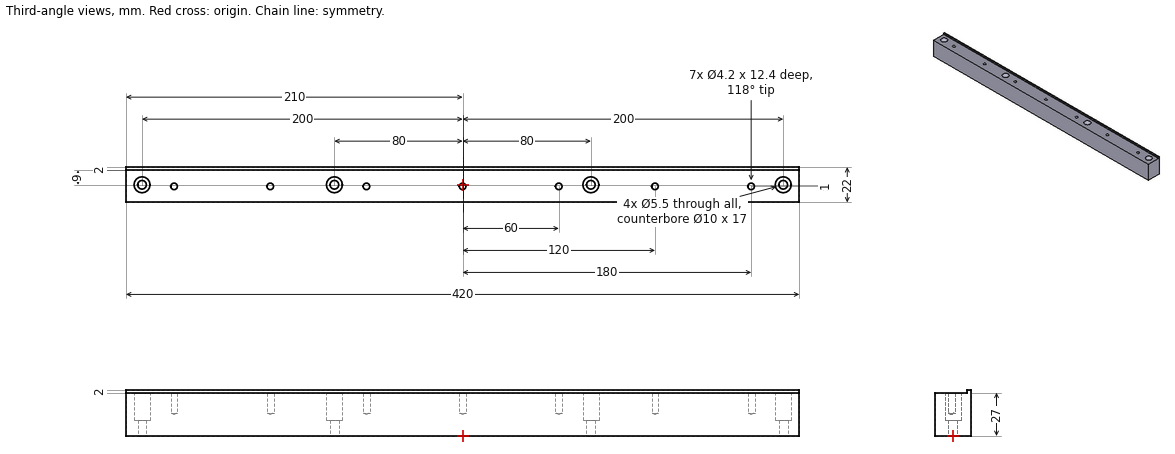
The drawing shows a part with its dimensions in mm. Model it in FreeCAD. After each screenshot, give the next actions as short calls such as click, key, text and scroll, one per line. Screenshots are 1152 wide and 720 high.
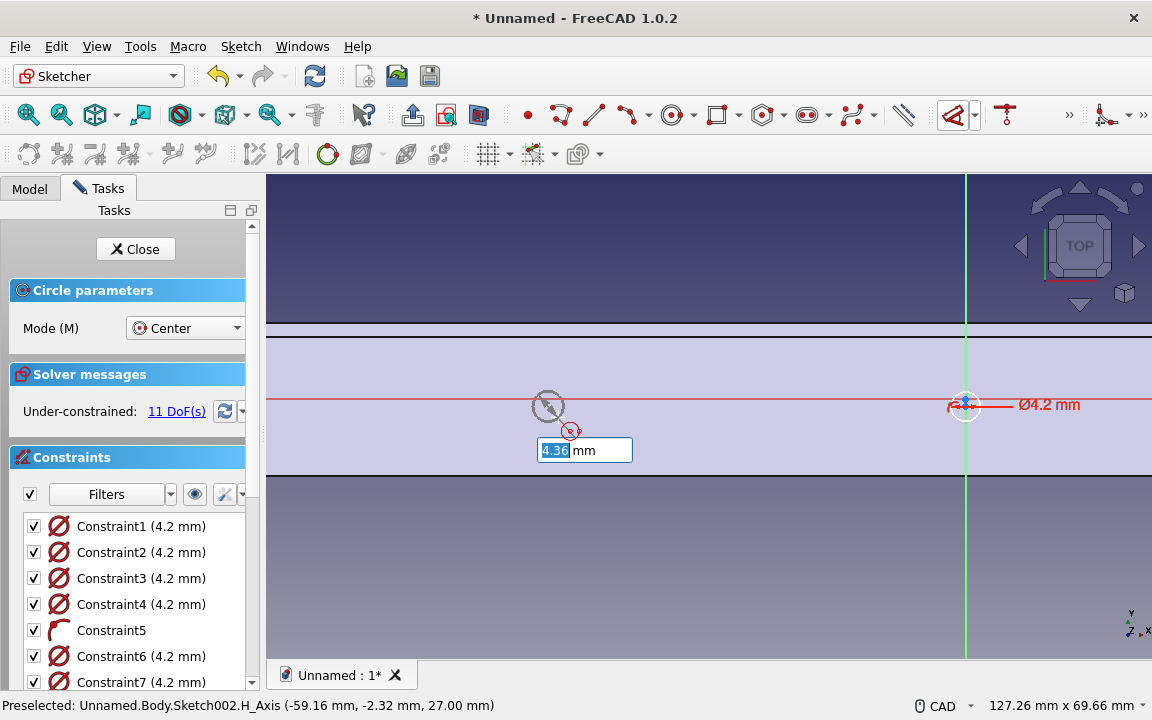
text(4.2)
key(Return)
key(Escape)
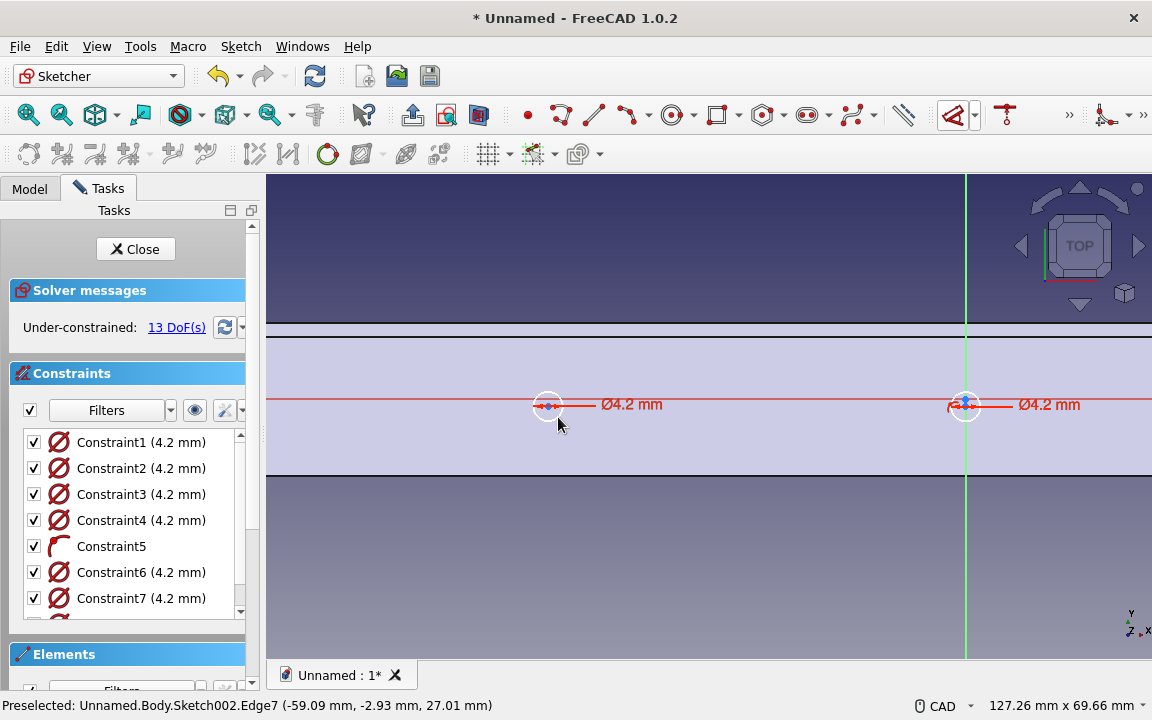
scroll(558, 419, down, 8)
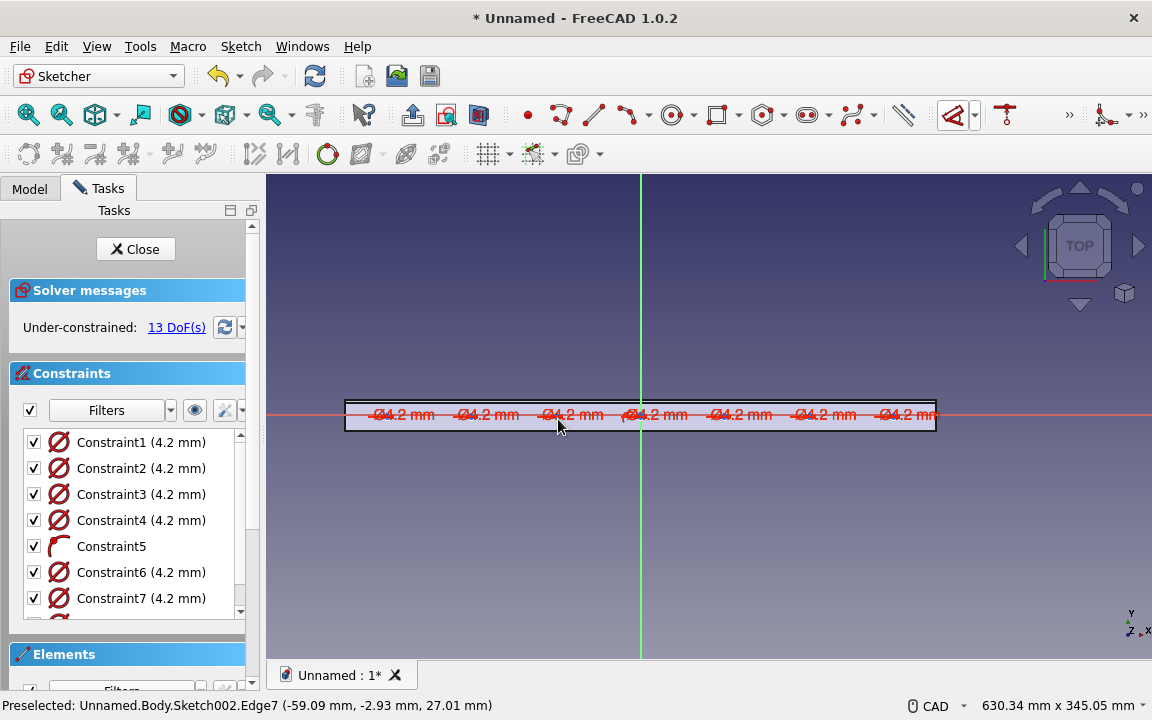
click(894, 417)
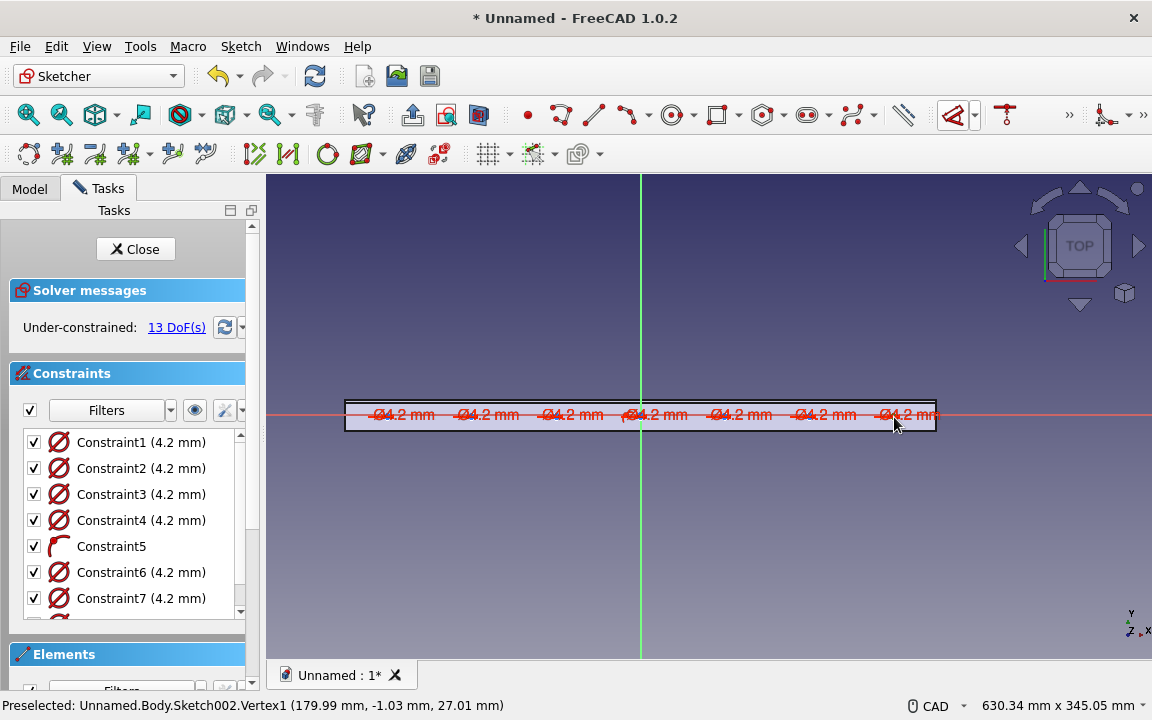
click(388, 417)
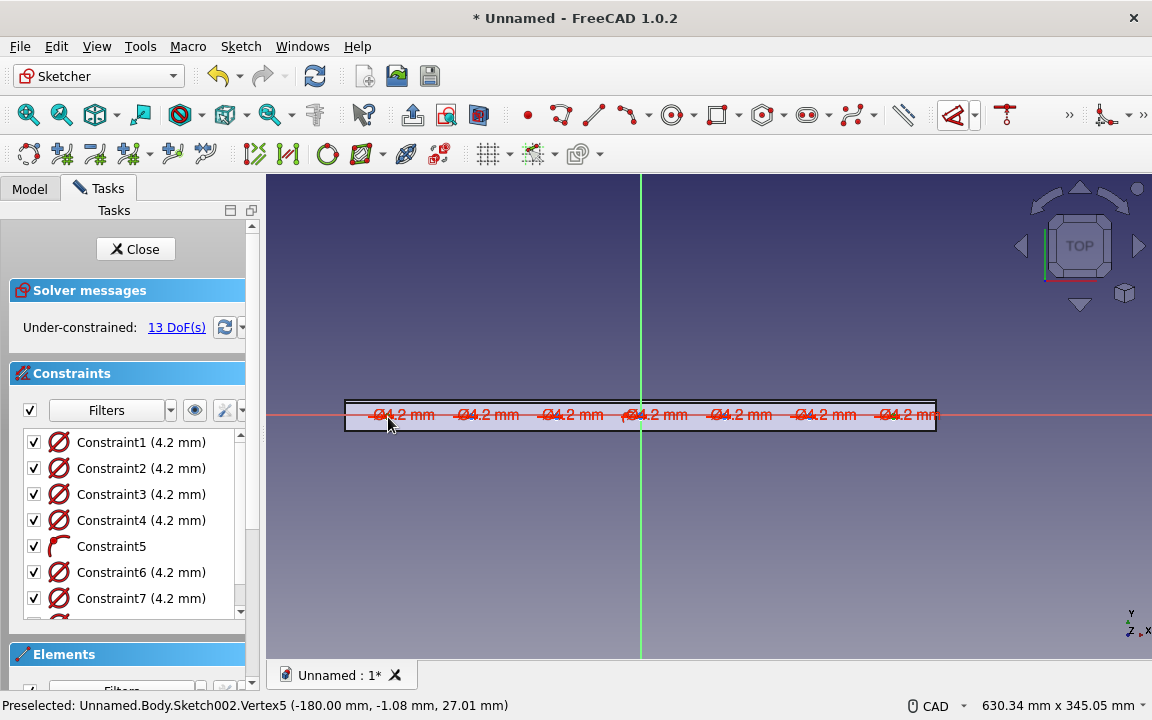
click(641, 600)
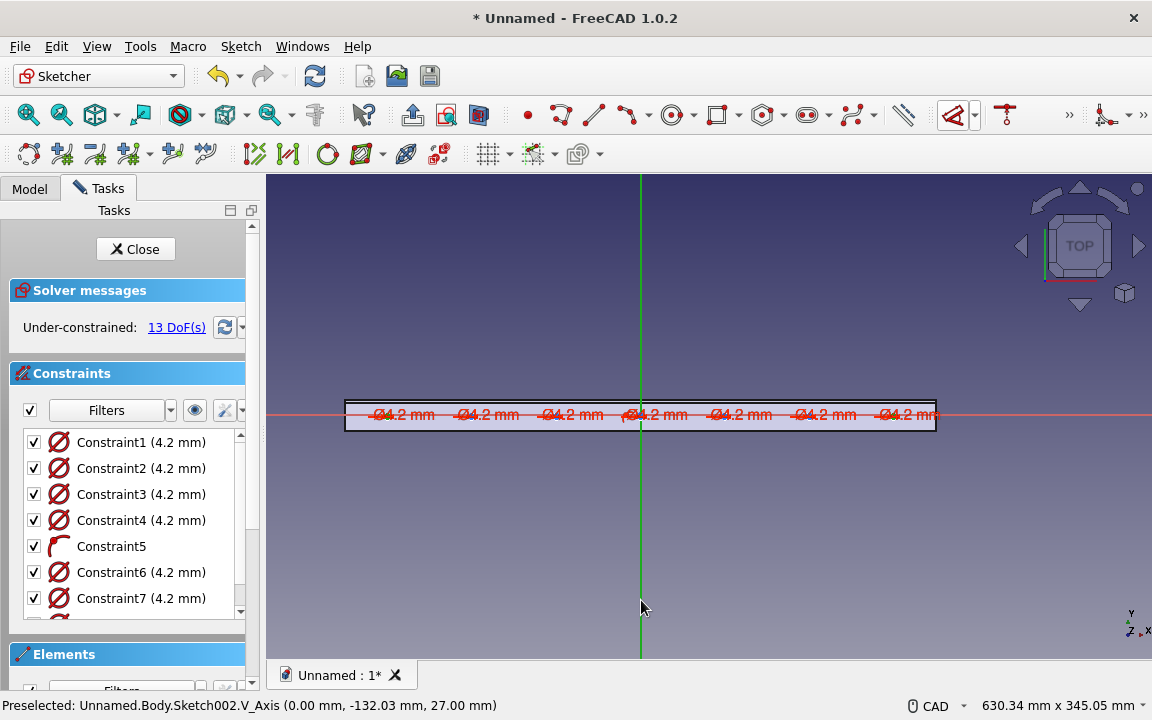
key(s)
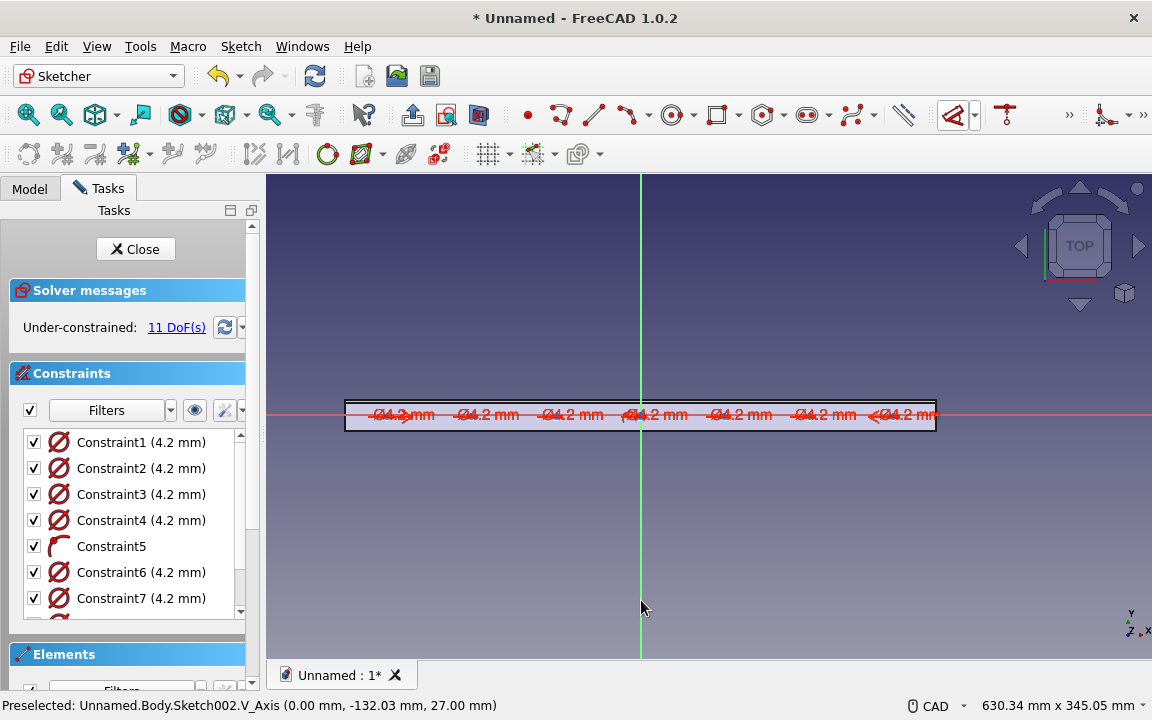
click(809, 417)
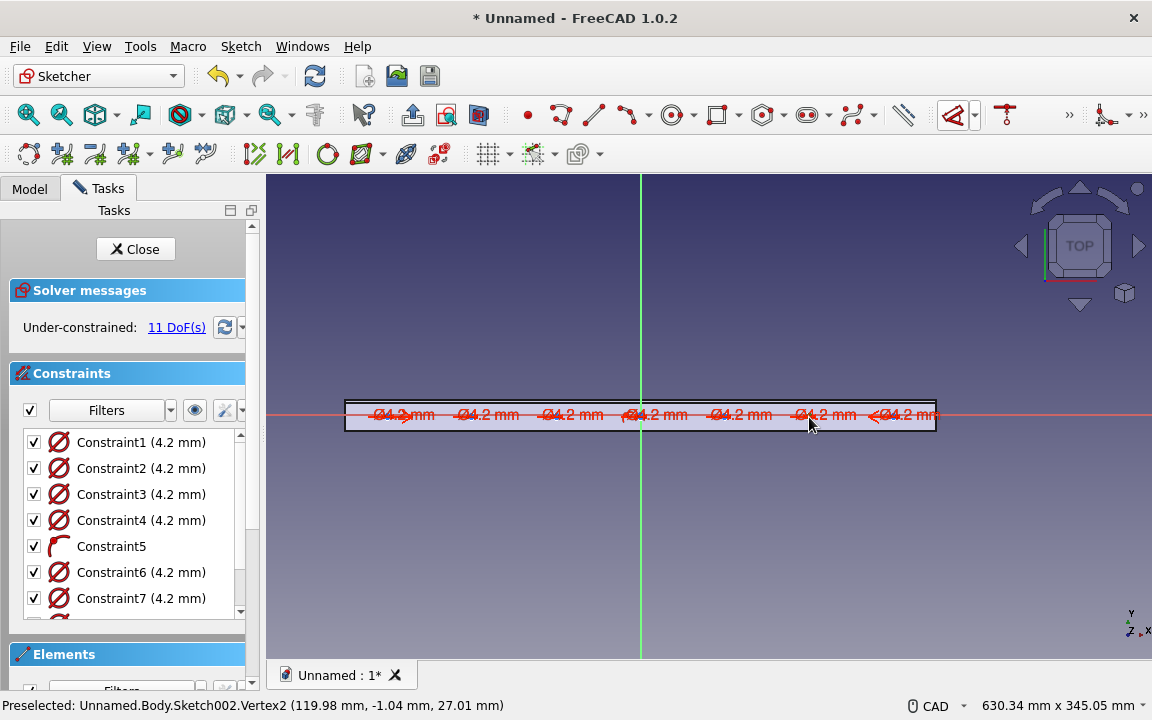
click(472, 417)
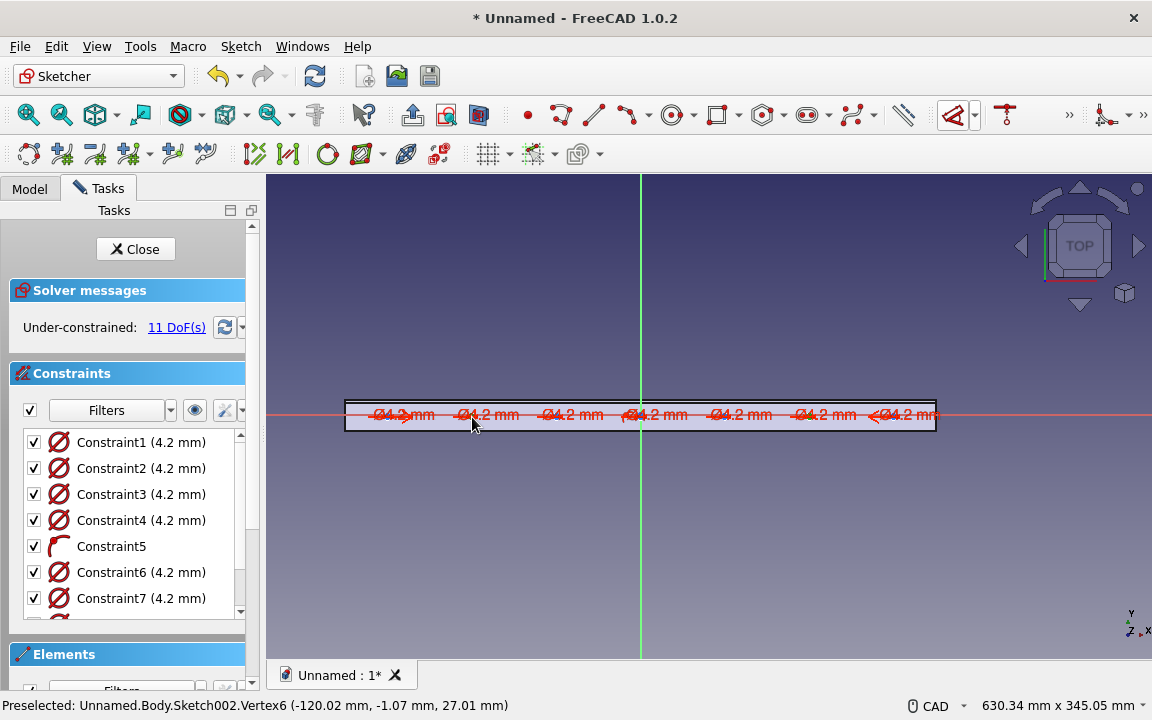
click(641, 600)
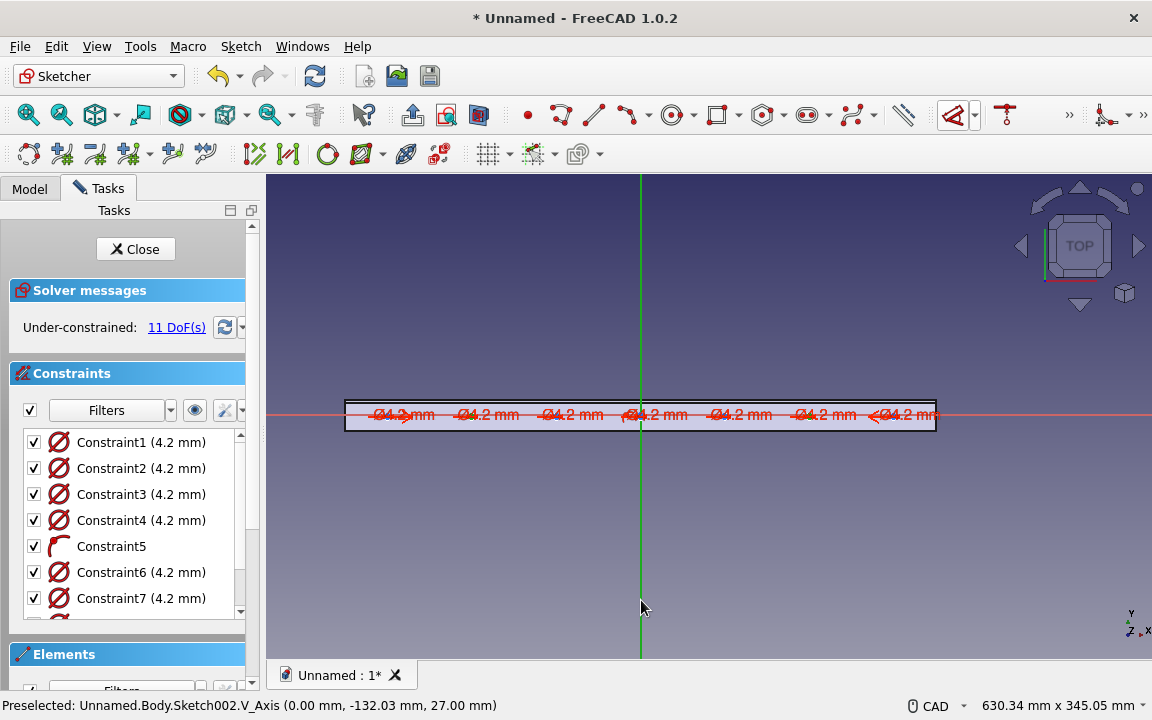
key(s)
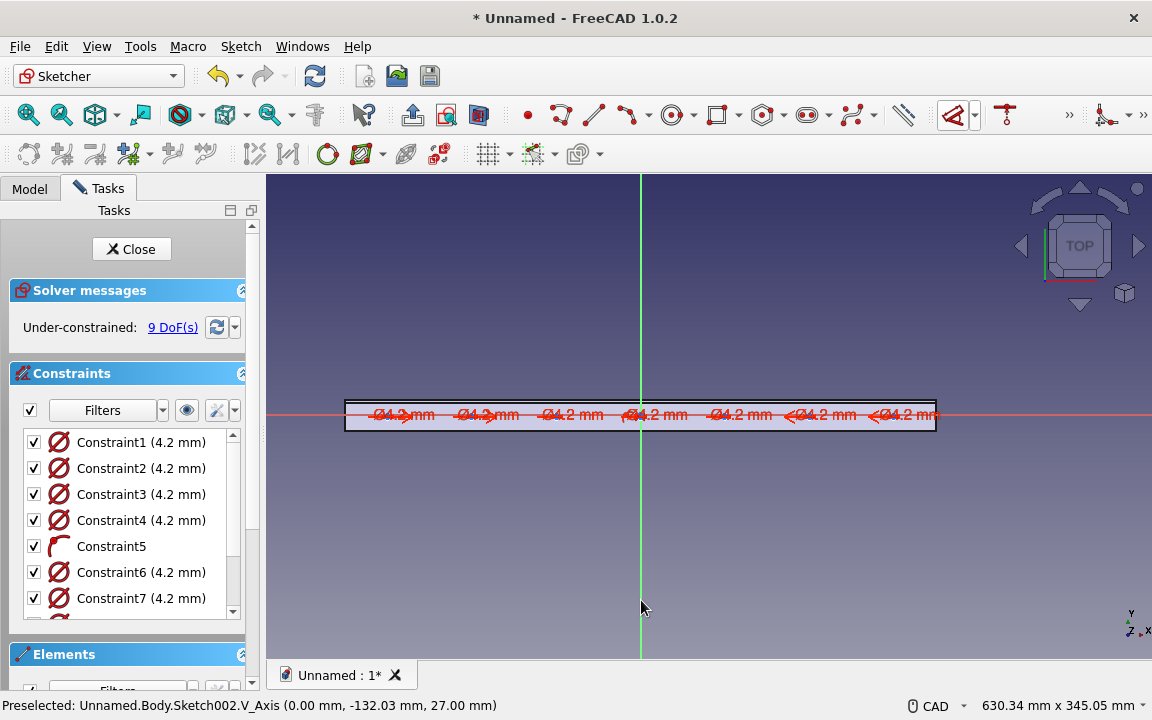
click(725, 417)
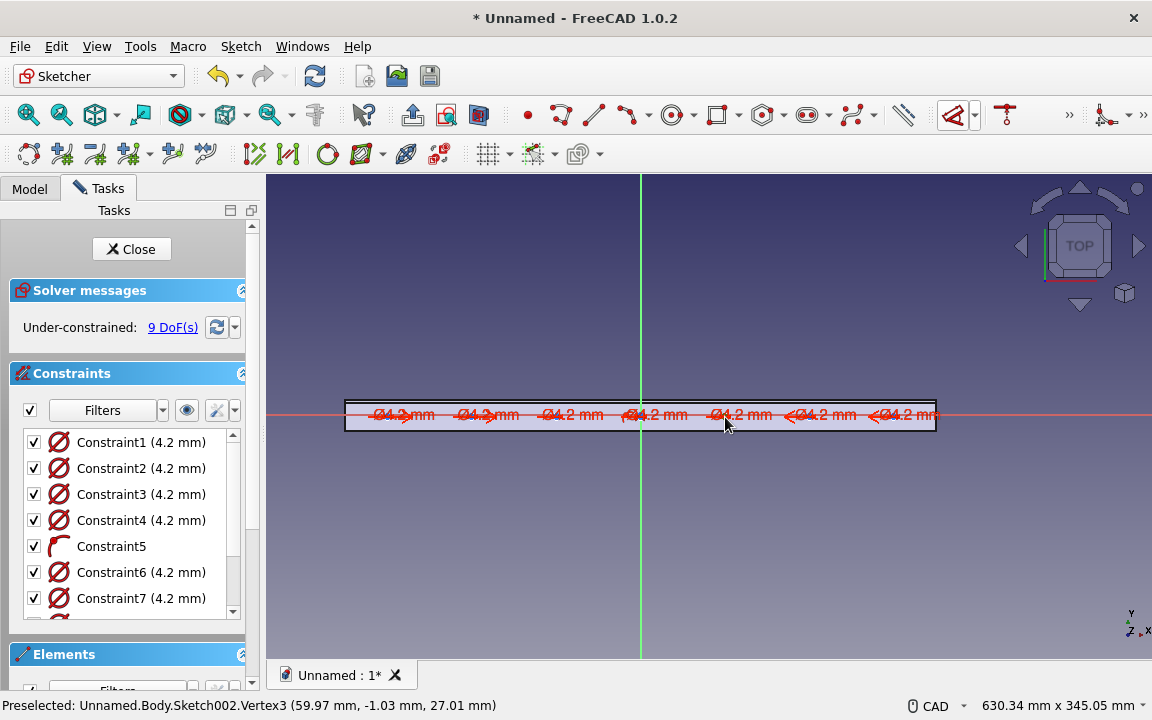
click(556, 417)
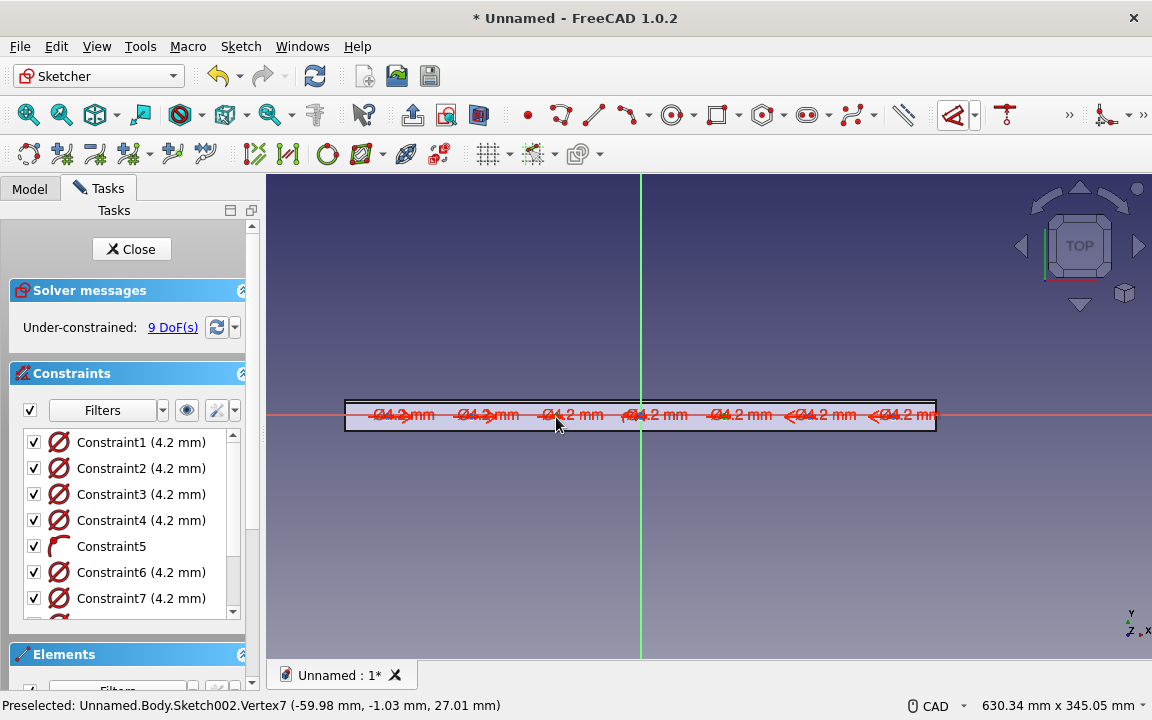
click(641, 600)